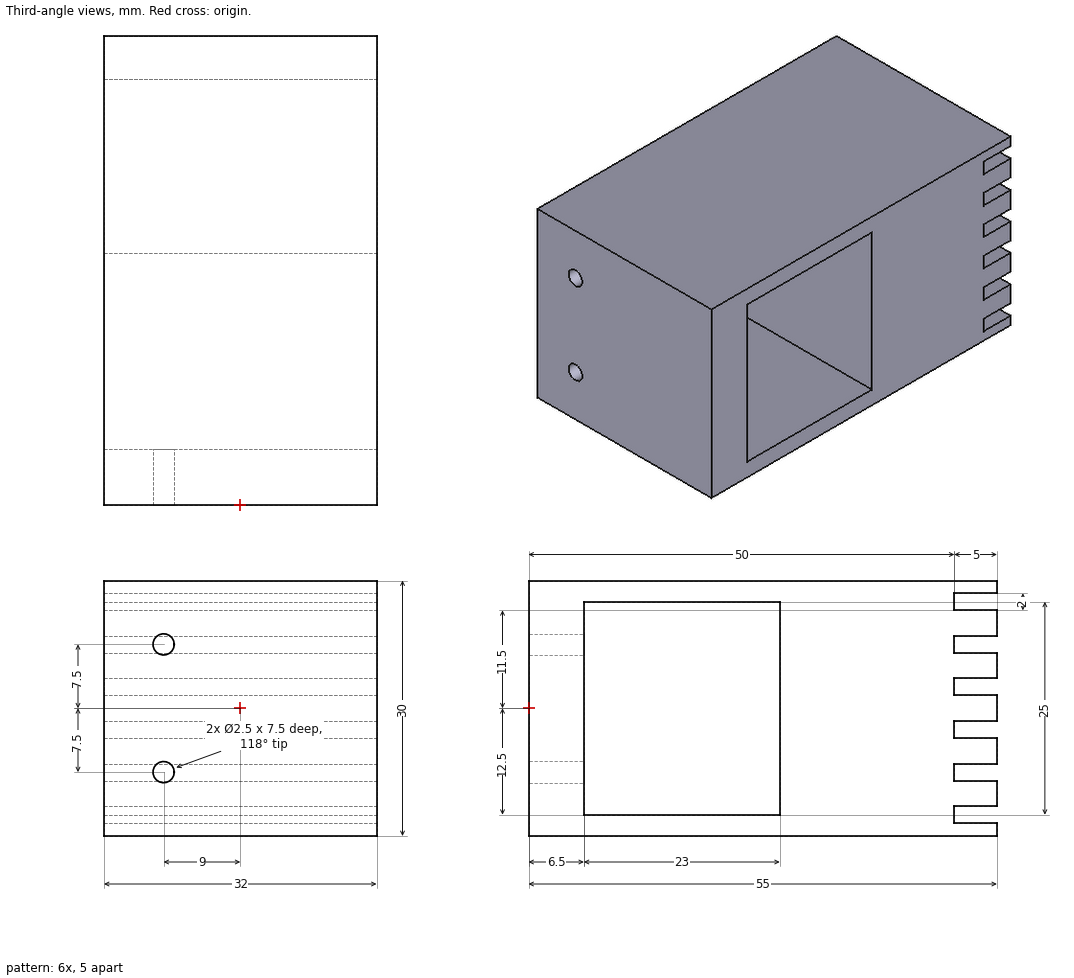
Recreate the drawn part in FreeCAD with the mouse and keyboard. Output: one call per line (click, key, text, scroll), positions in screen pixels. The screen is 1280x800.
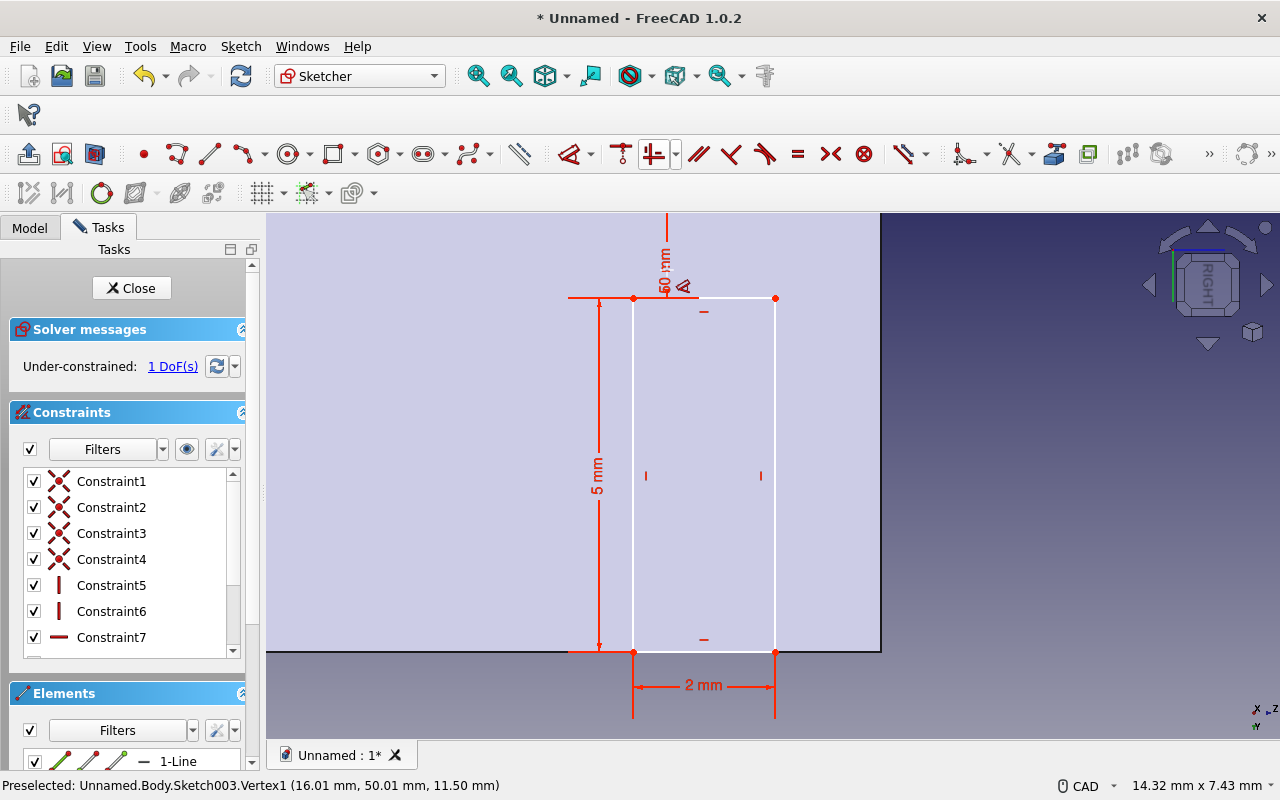
click(633, 298)
click(464, 332)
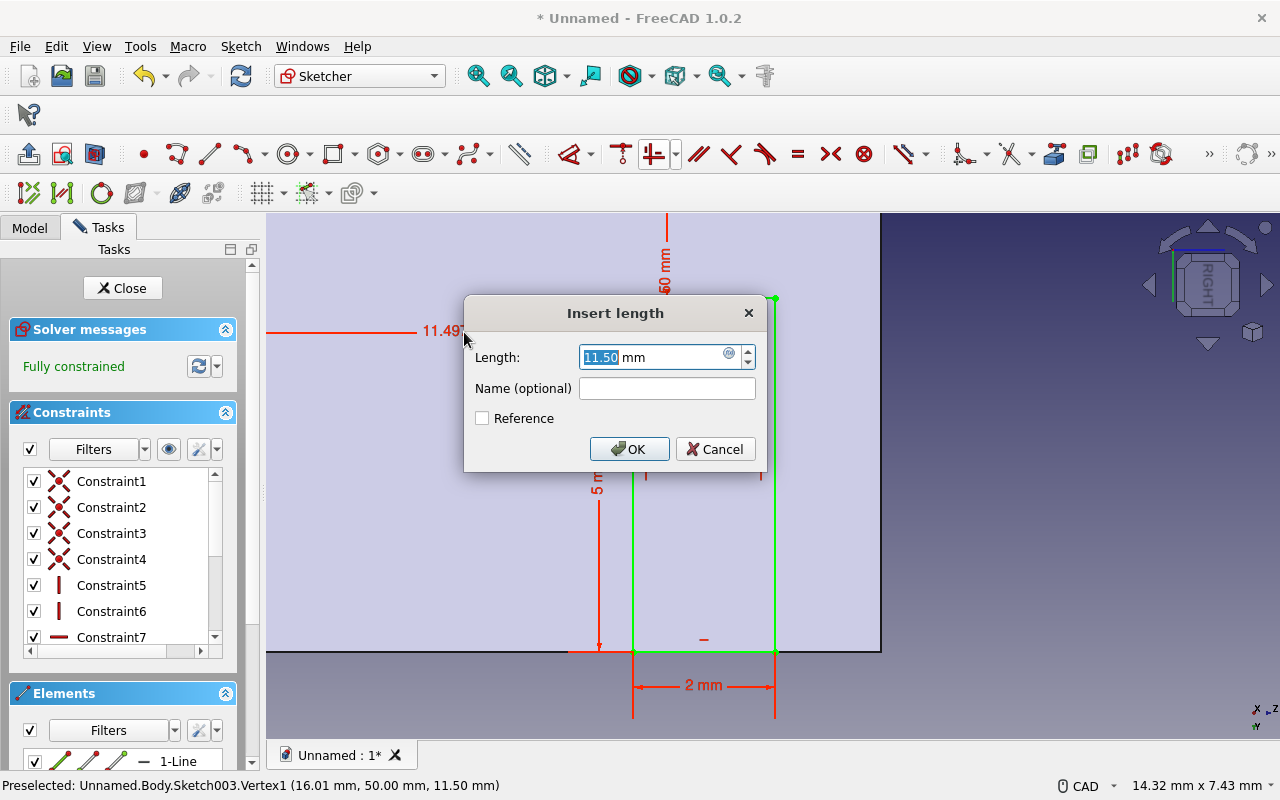
text(11.5)
key(Return)
key(Escape)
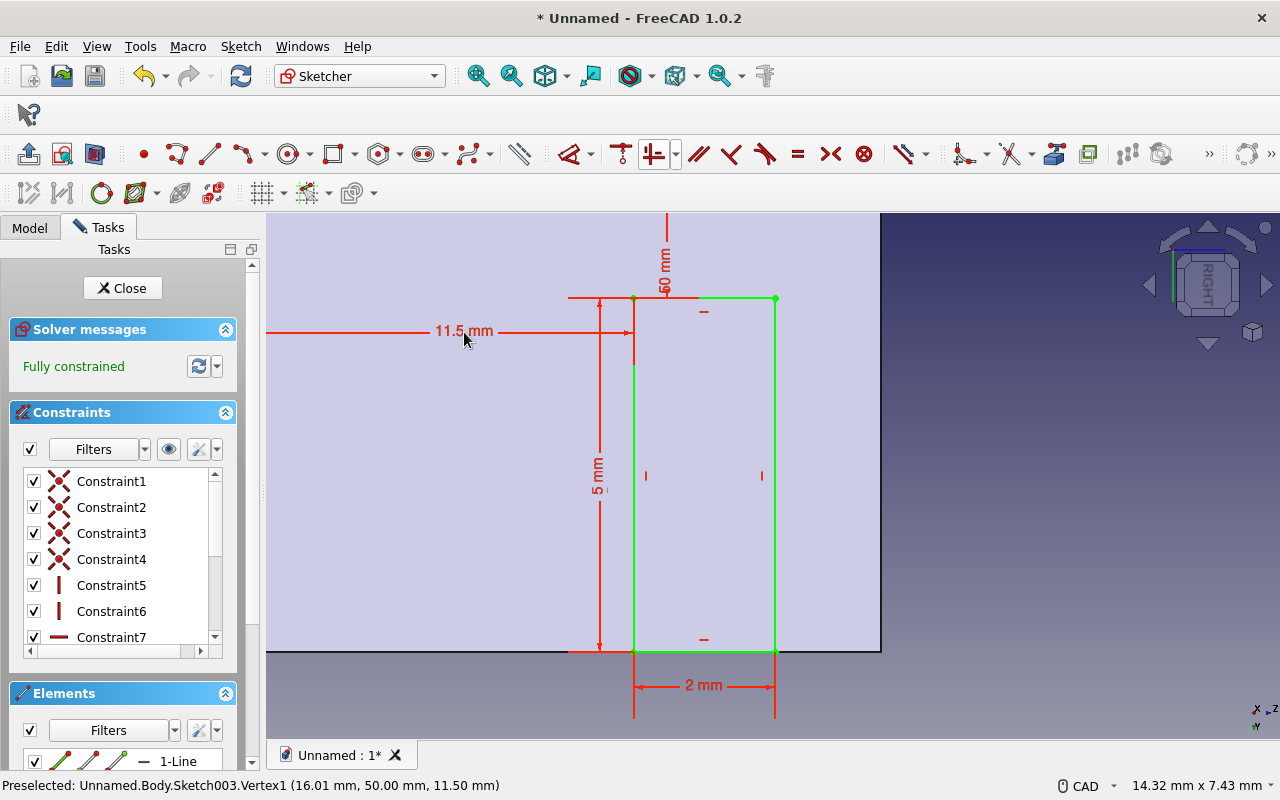
click(123, 288)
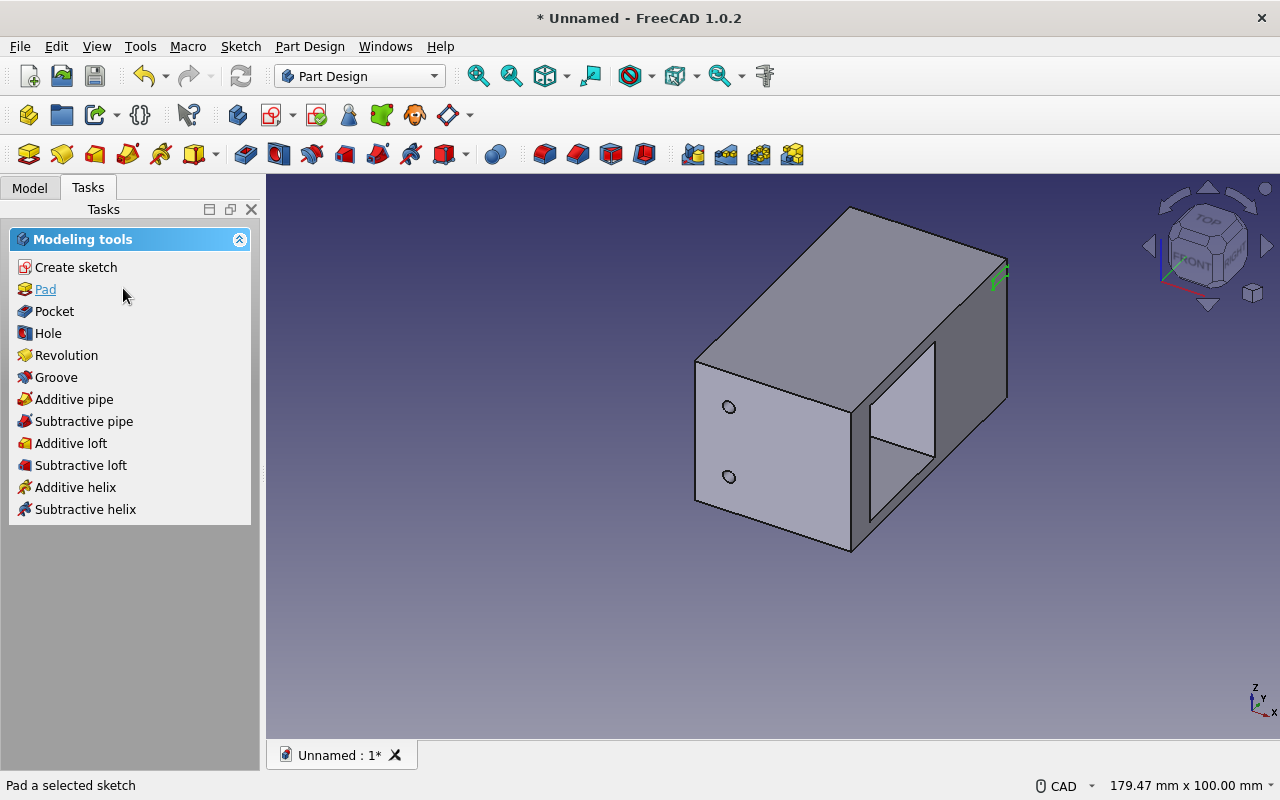
click(246, 154)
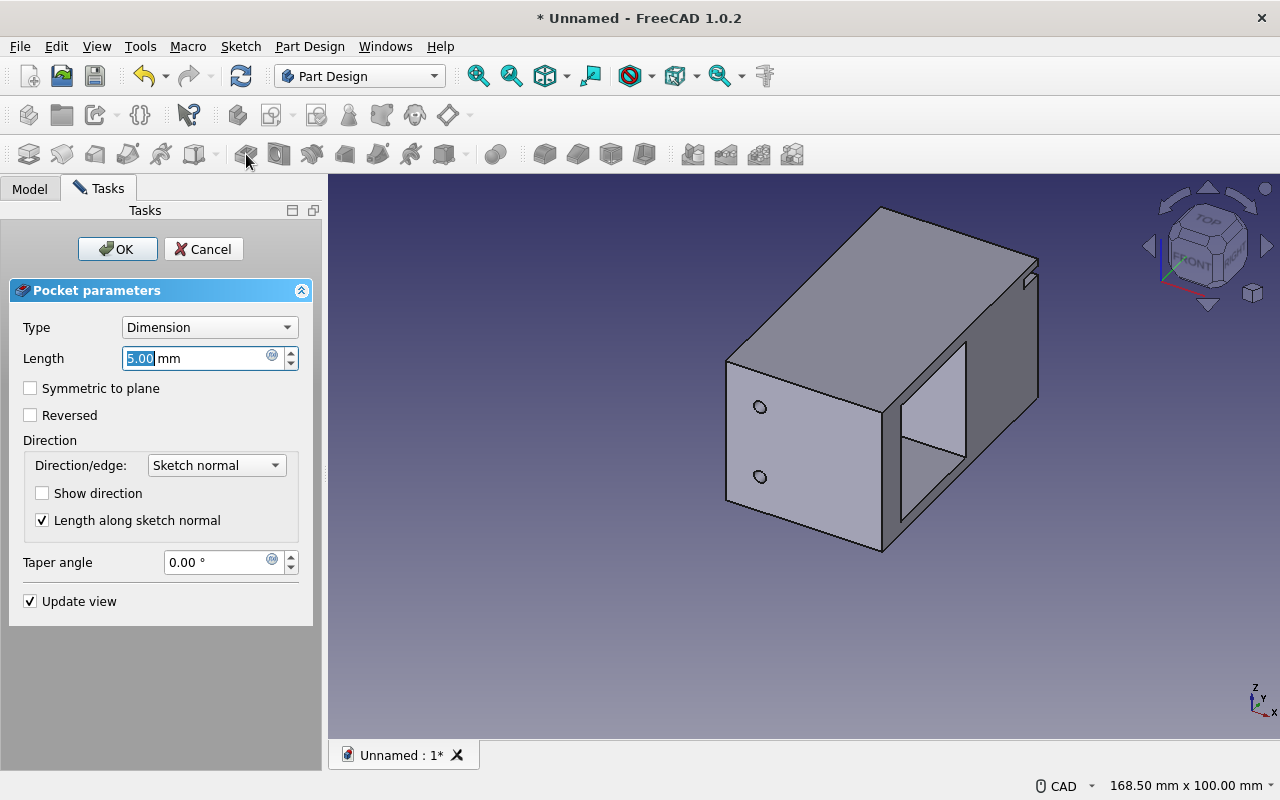
click(210, 328)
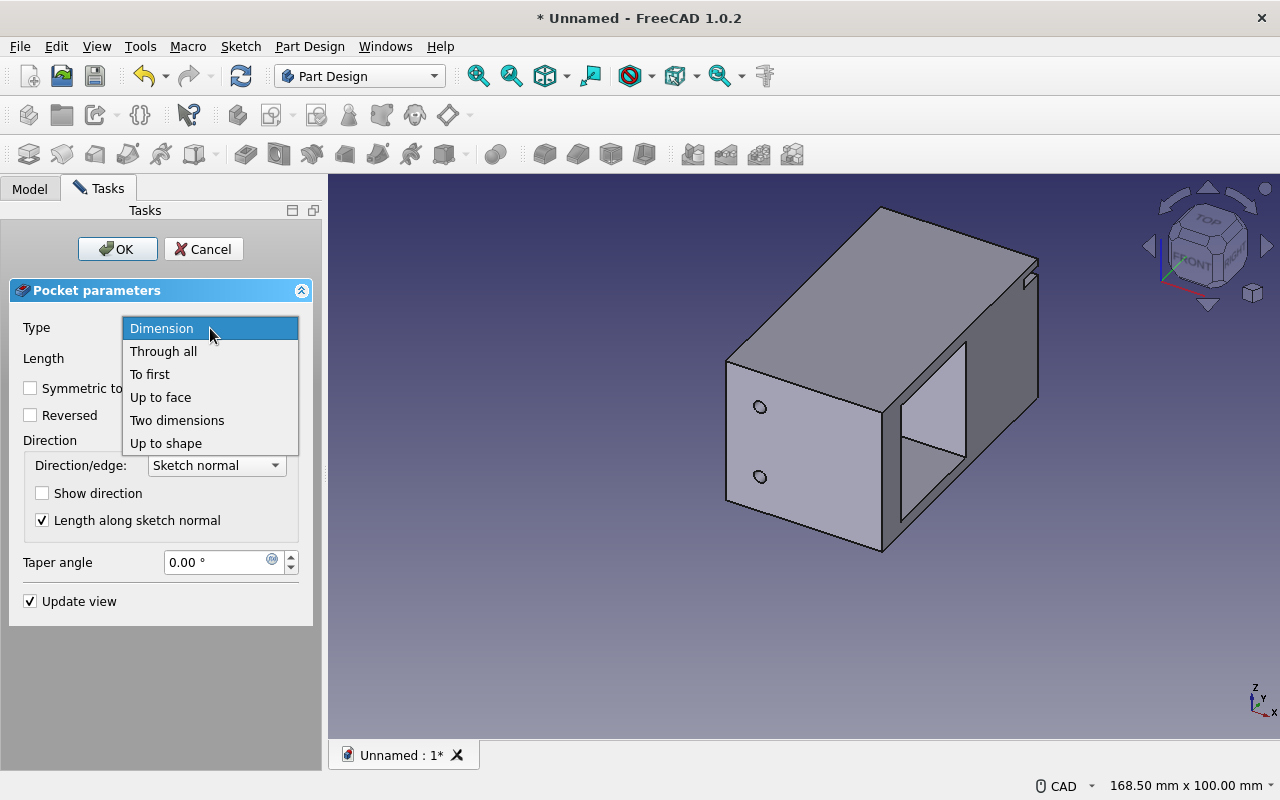
click(208, 352)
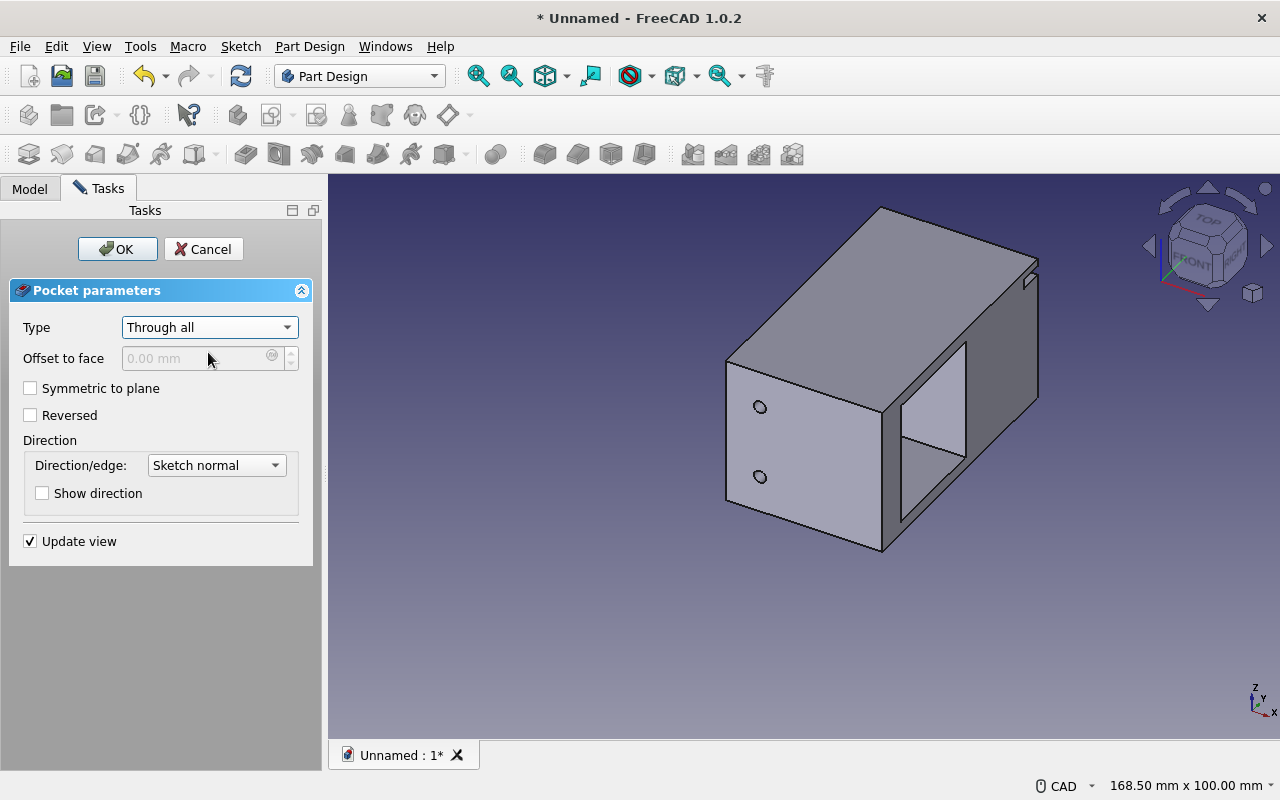
click(118, 249)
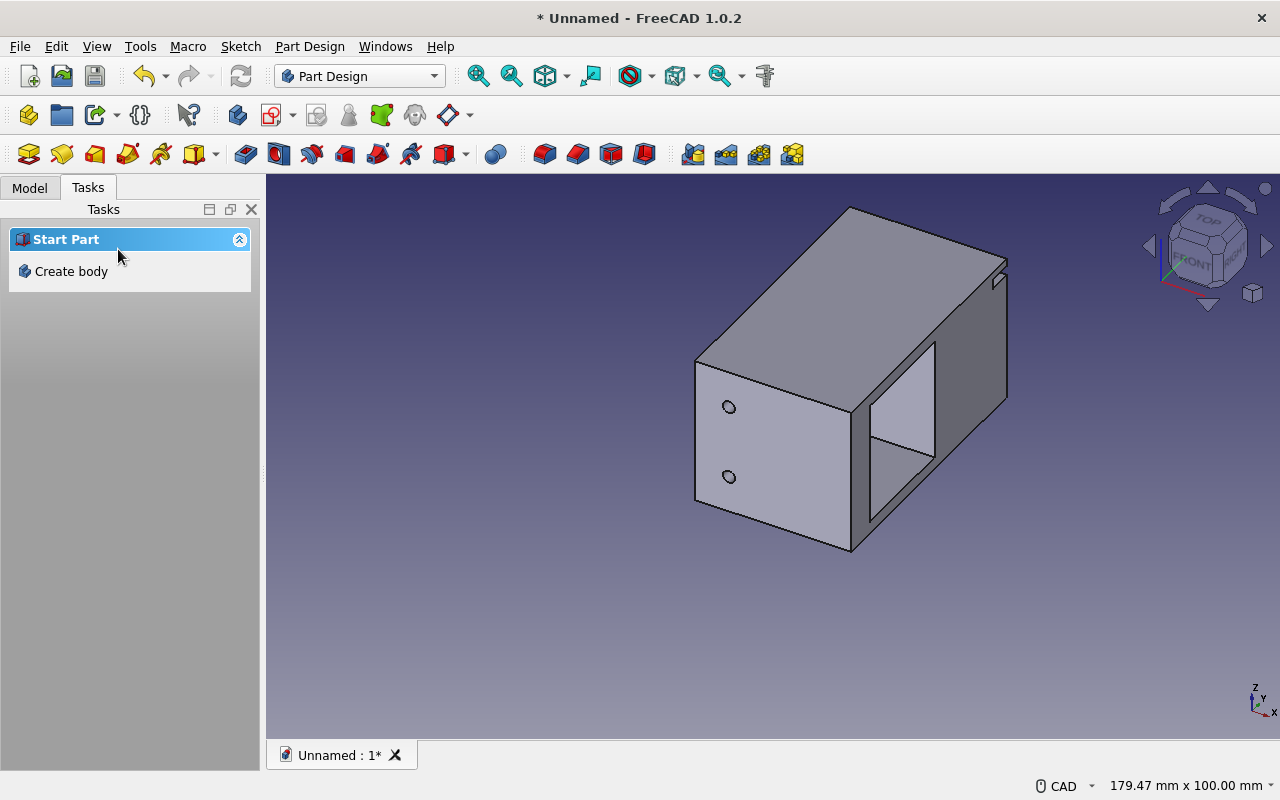
click(30, 188)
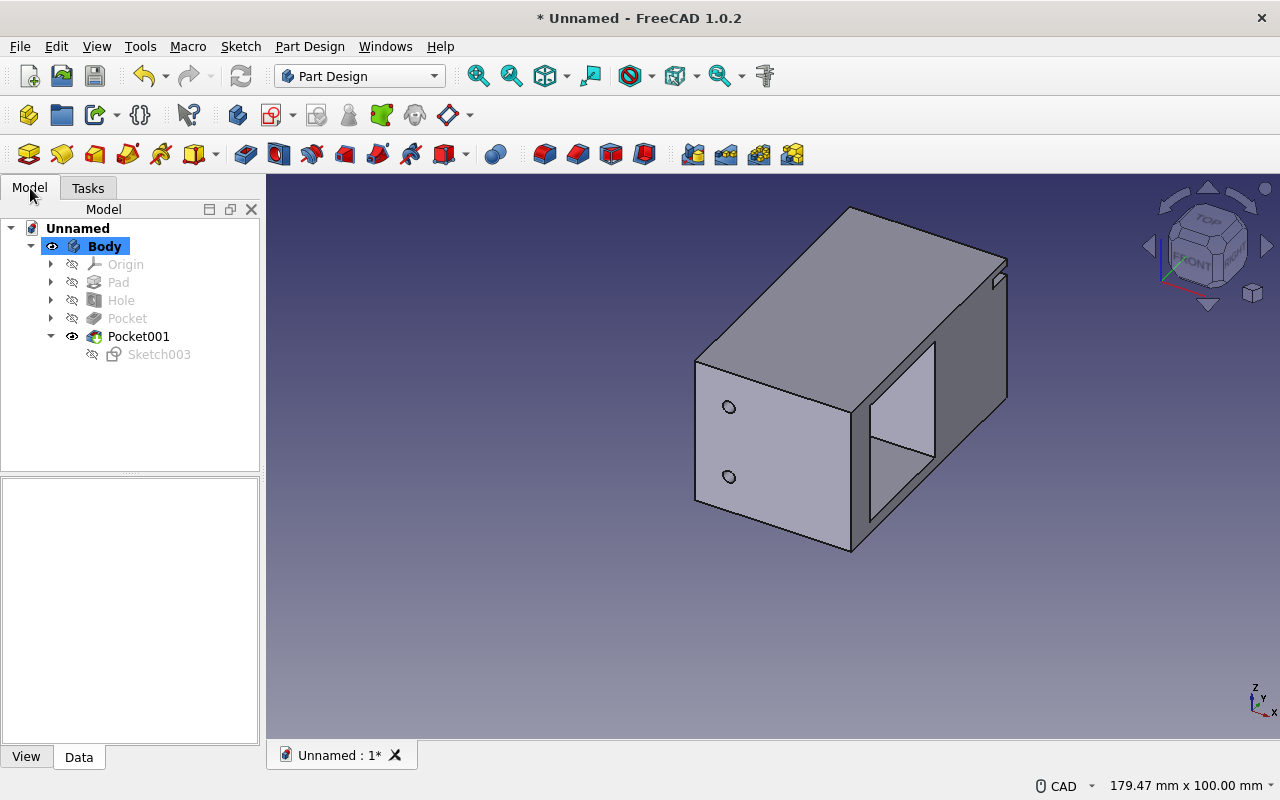
click(117, 336)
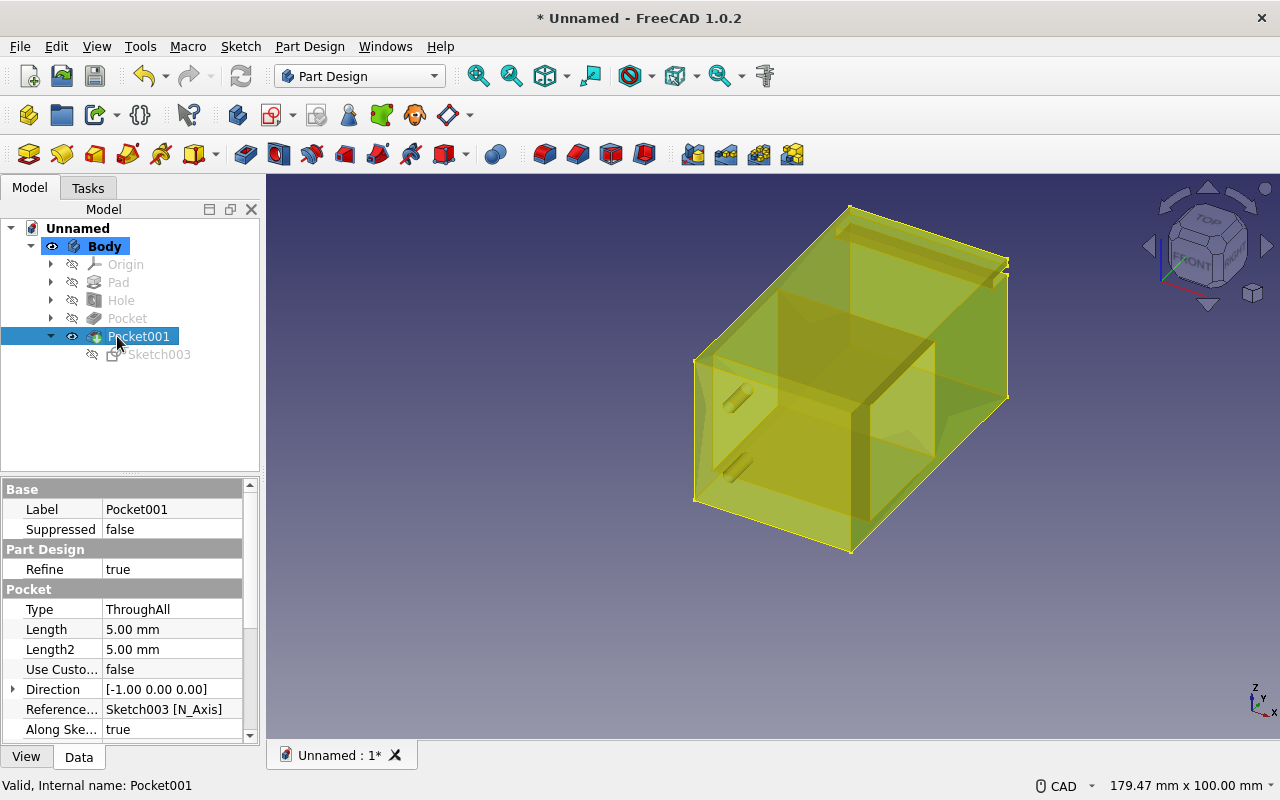
click(726, 154)